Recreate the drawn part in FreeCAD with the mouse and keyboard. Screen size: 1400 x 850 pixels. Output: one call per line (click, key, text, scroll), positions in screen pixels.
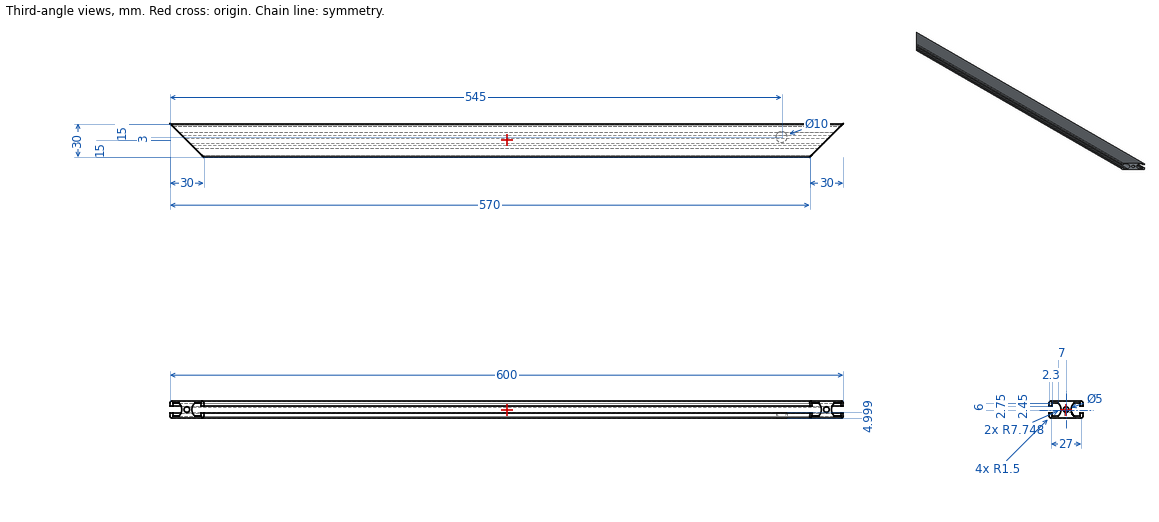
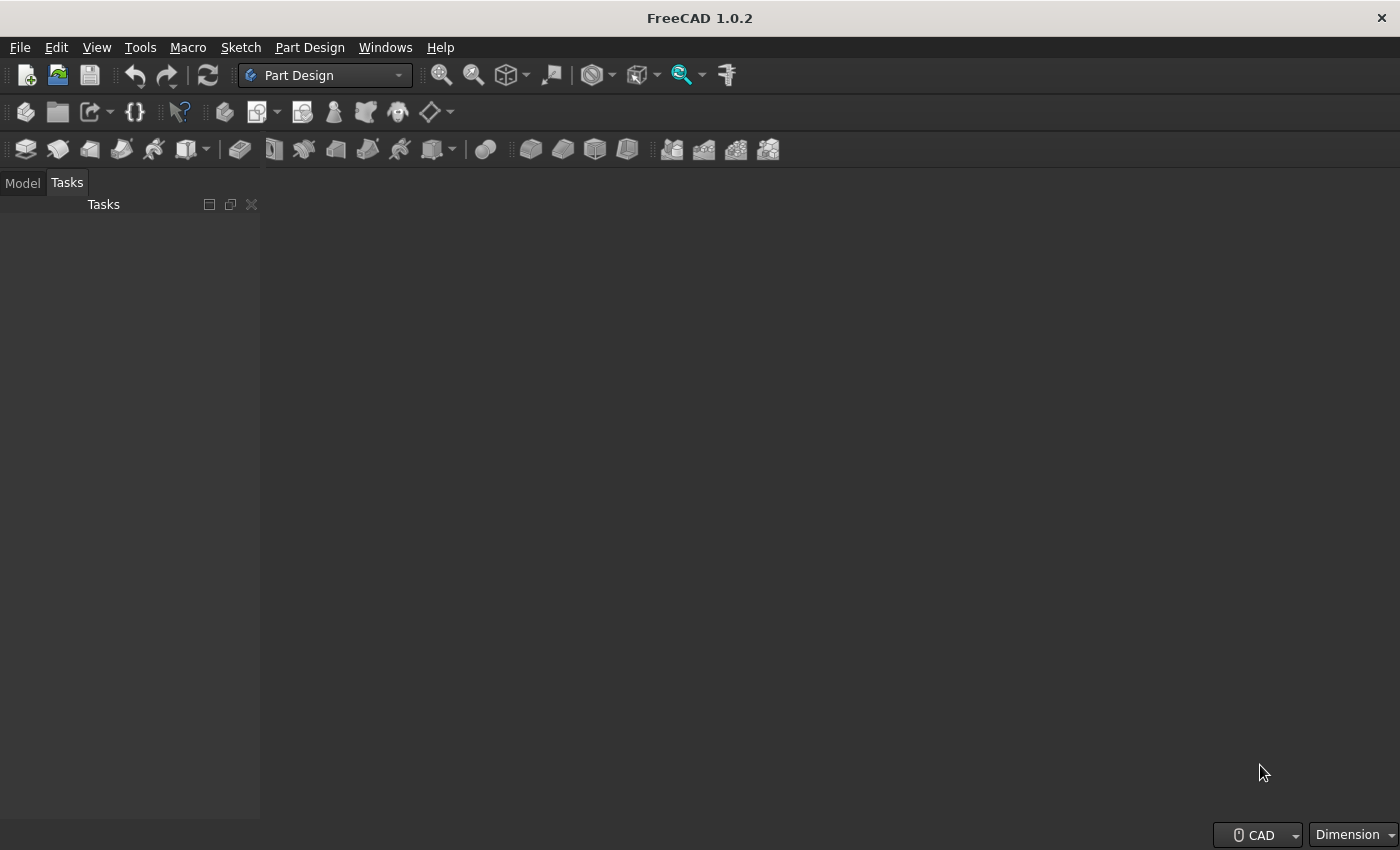
key(ctrl+n)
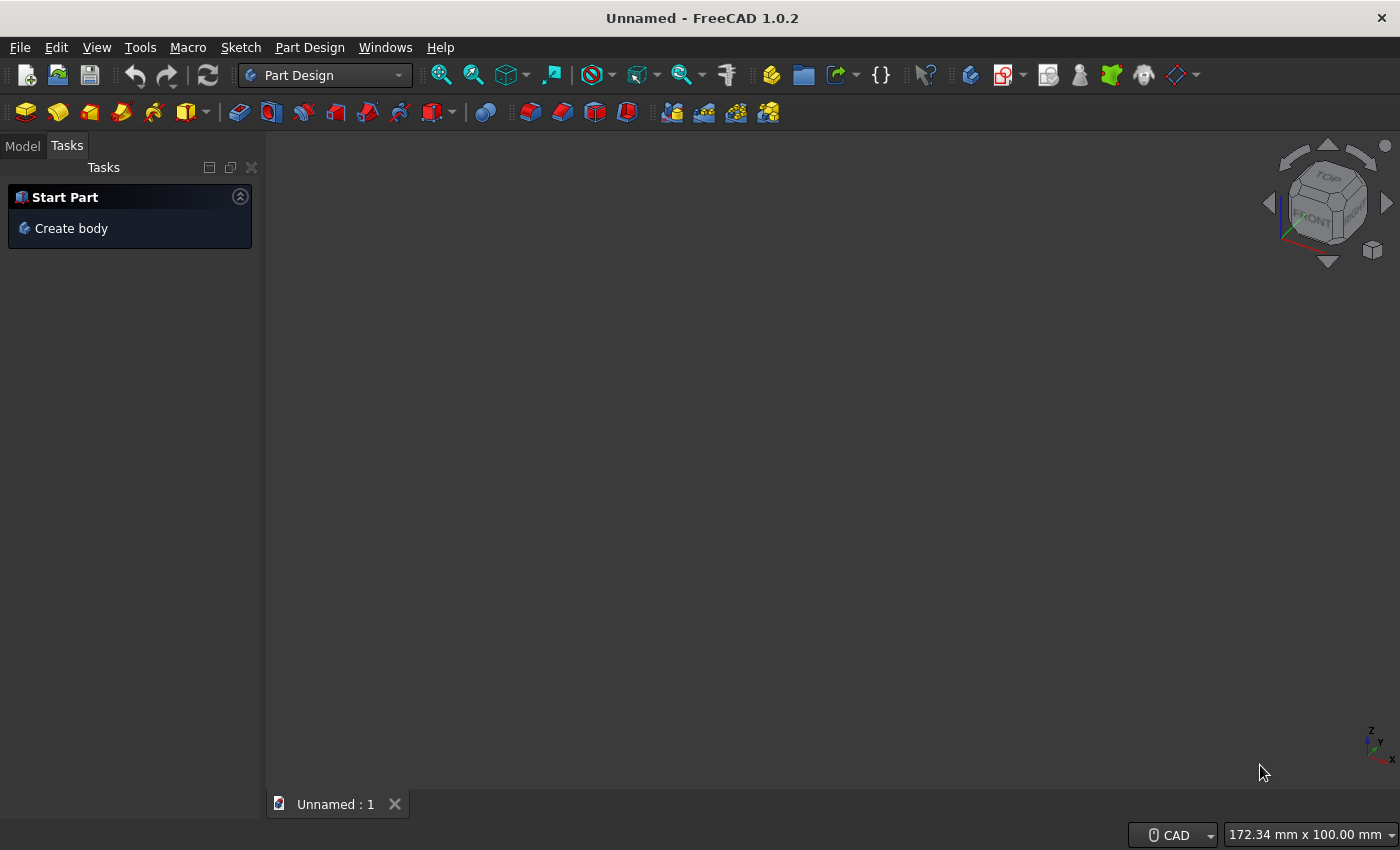
click(972, 76)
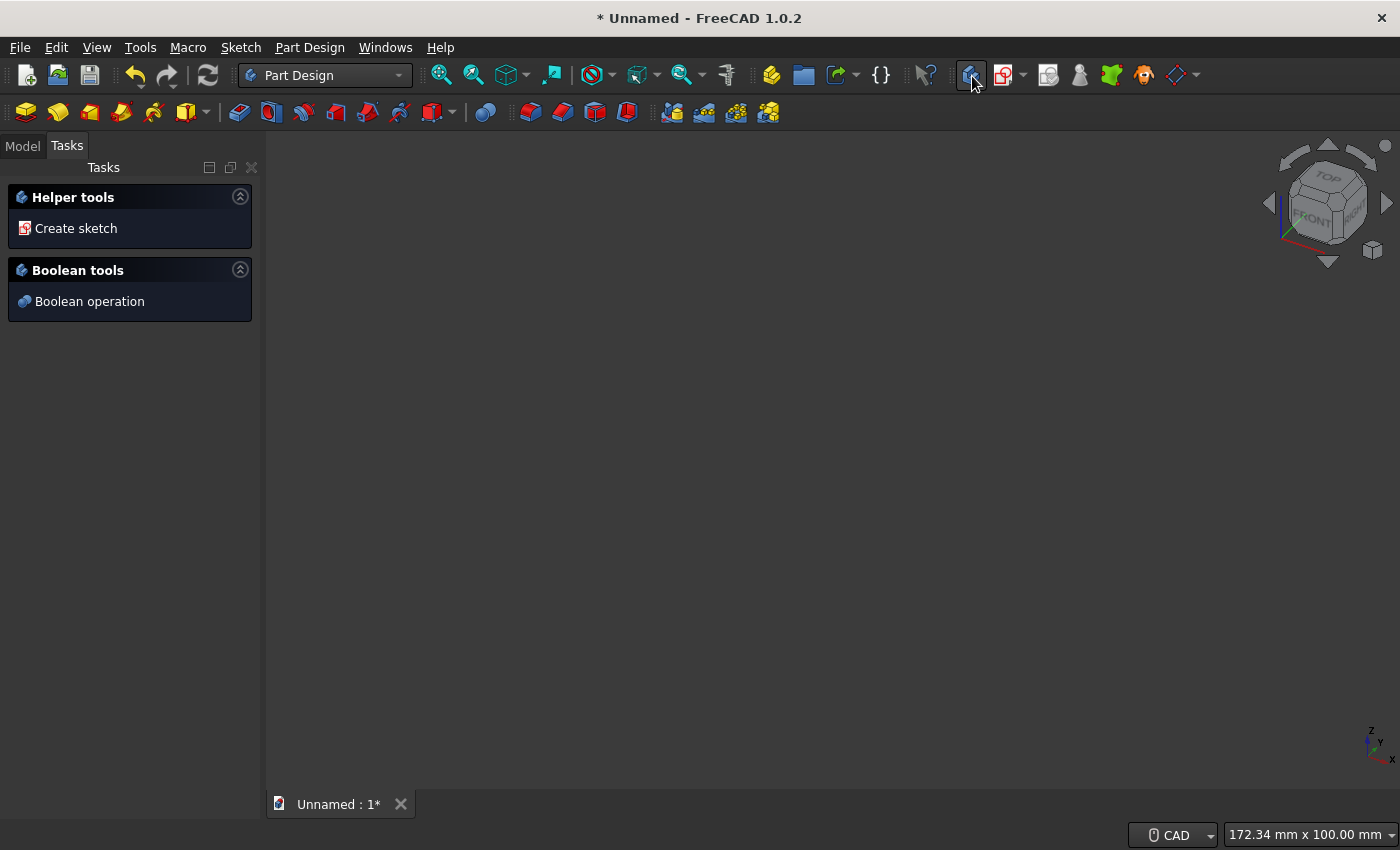
click(23, 145)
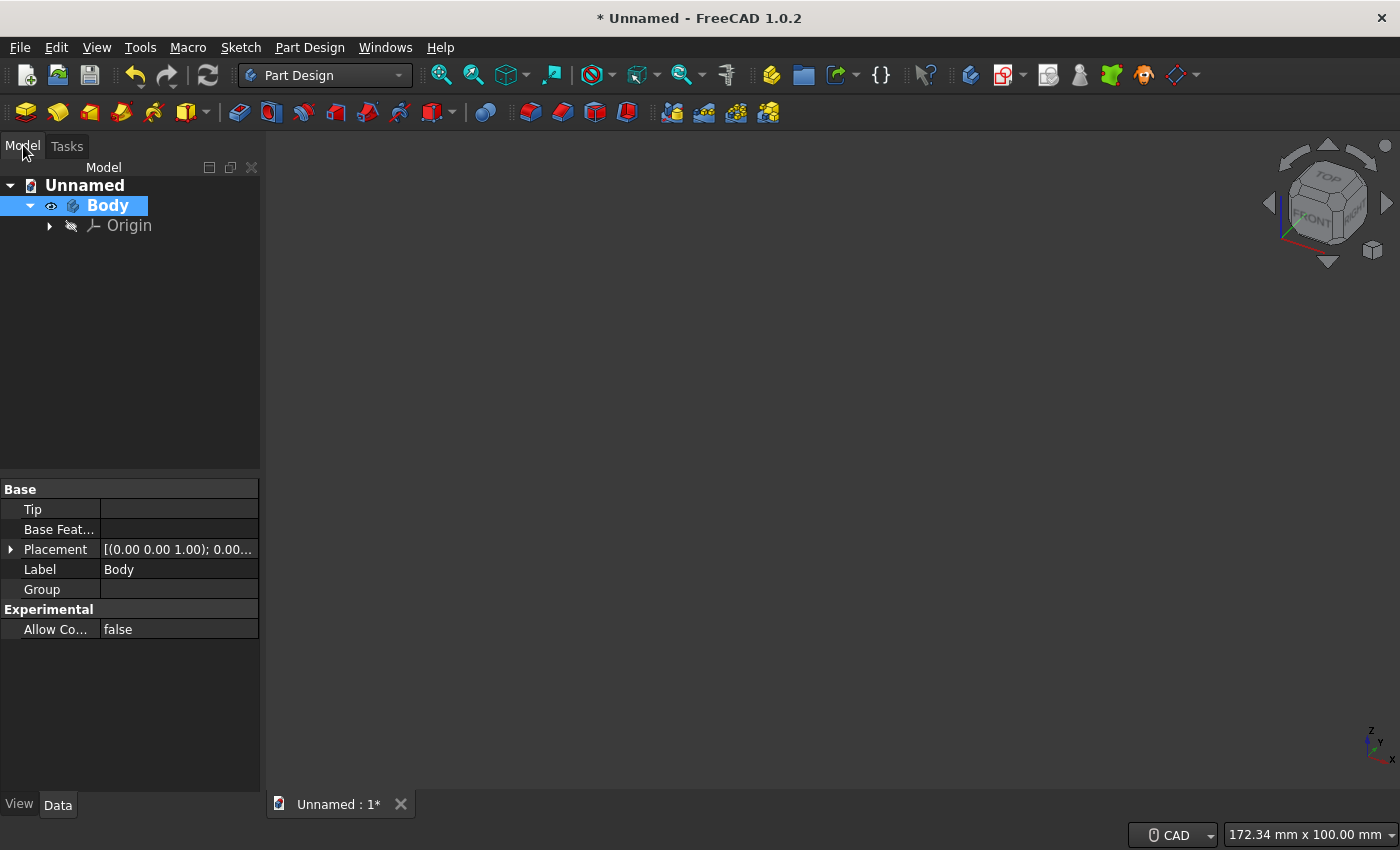
click(50, 226)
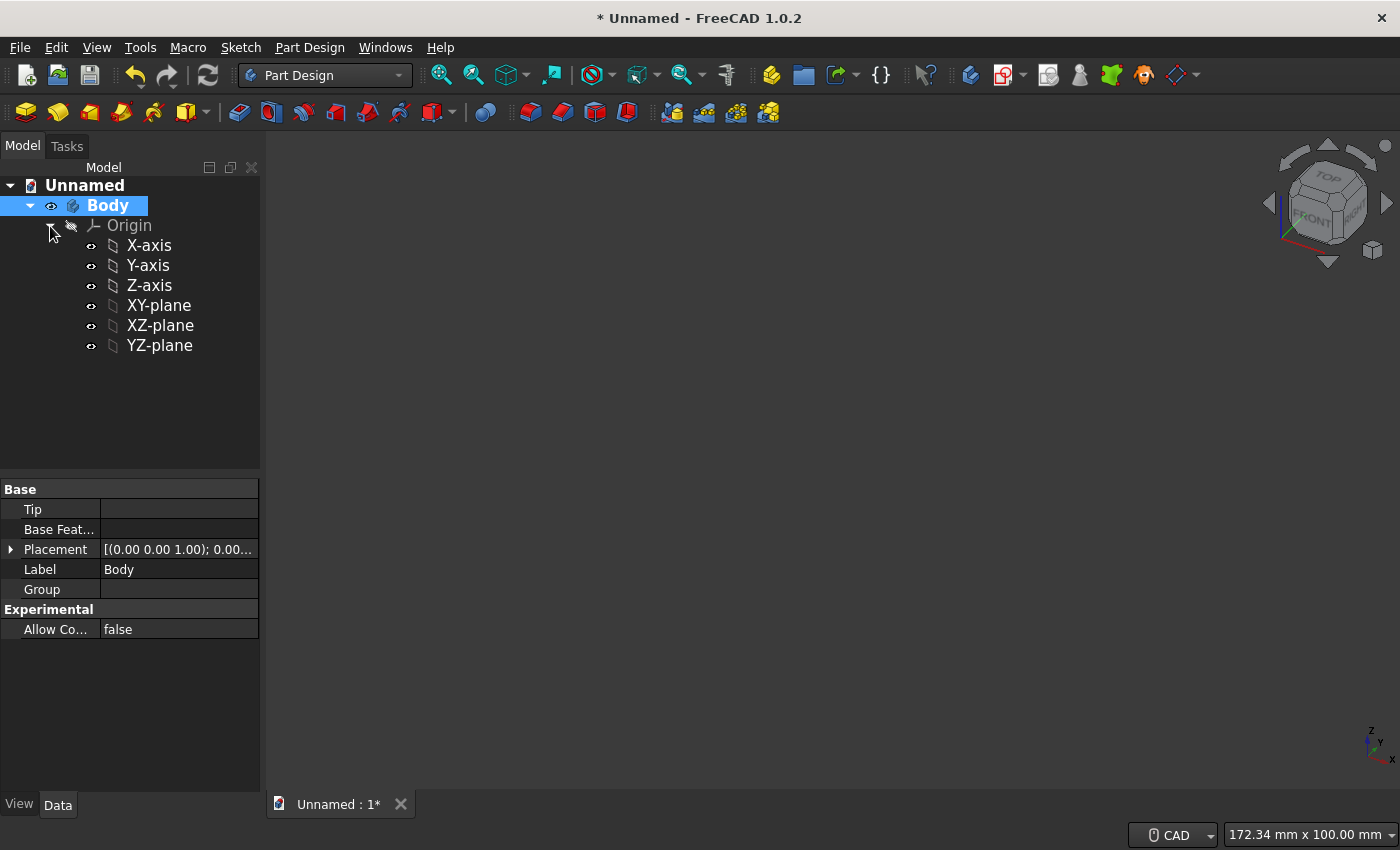
click(136, 346)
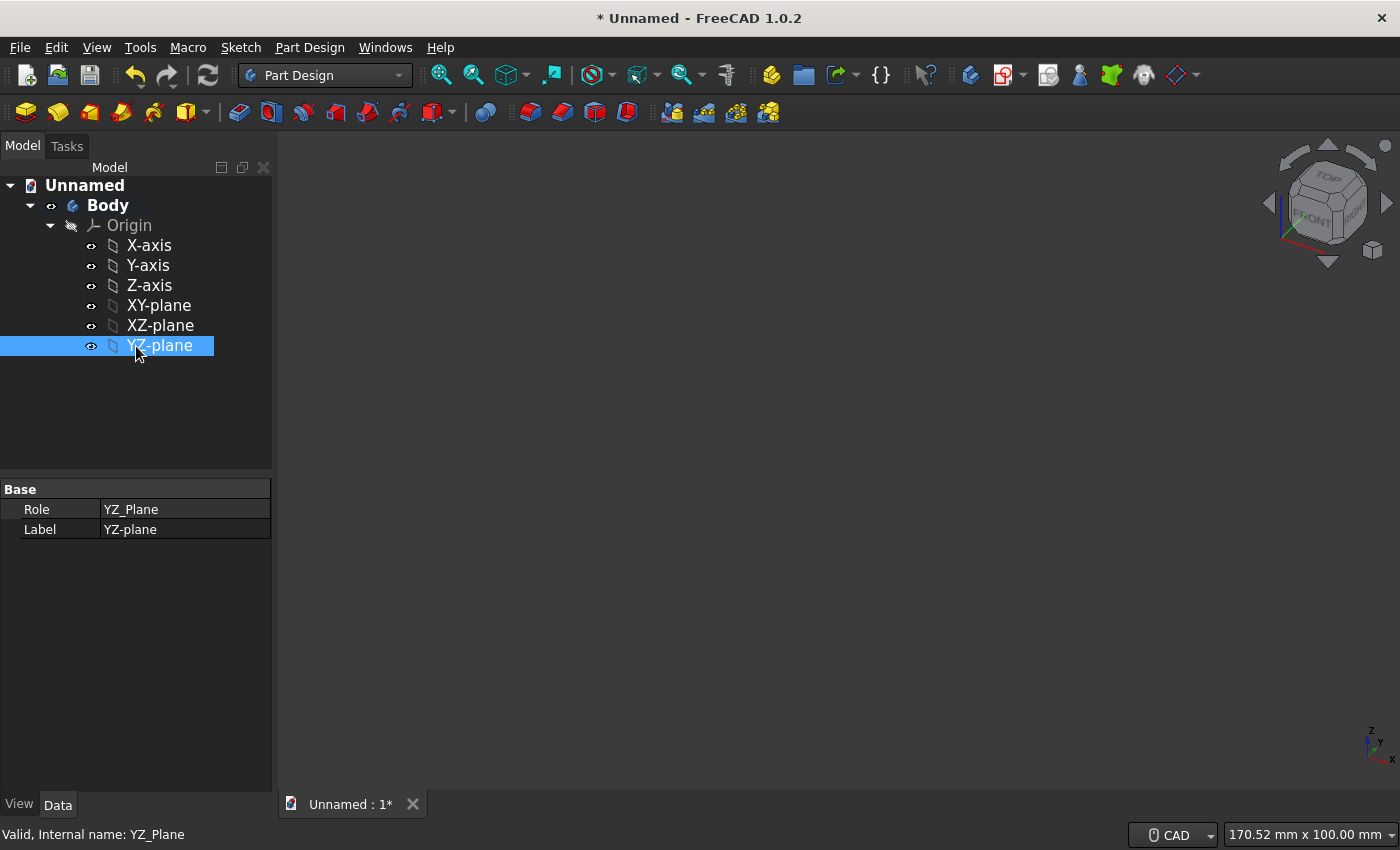
click(1176, 76)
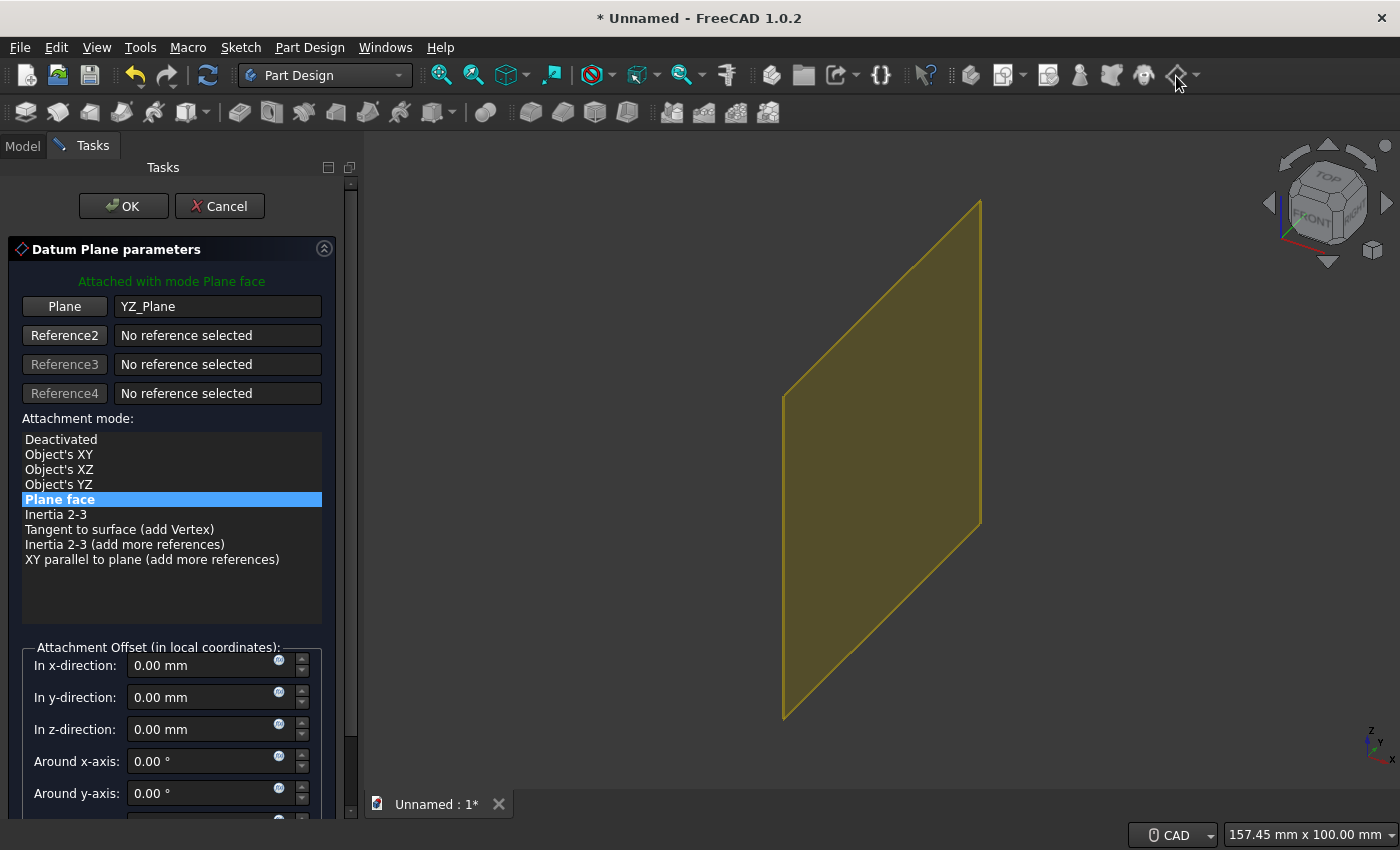
triple_click(210, 729)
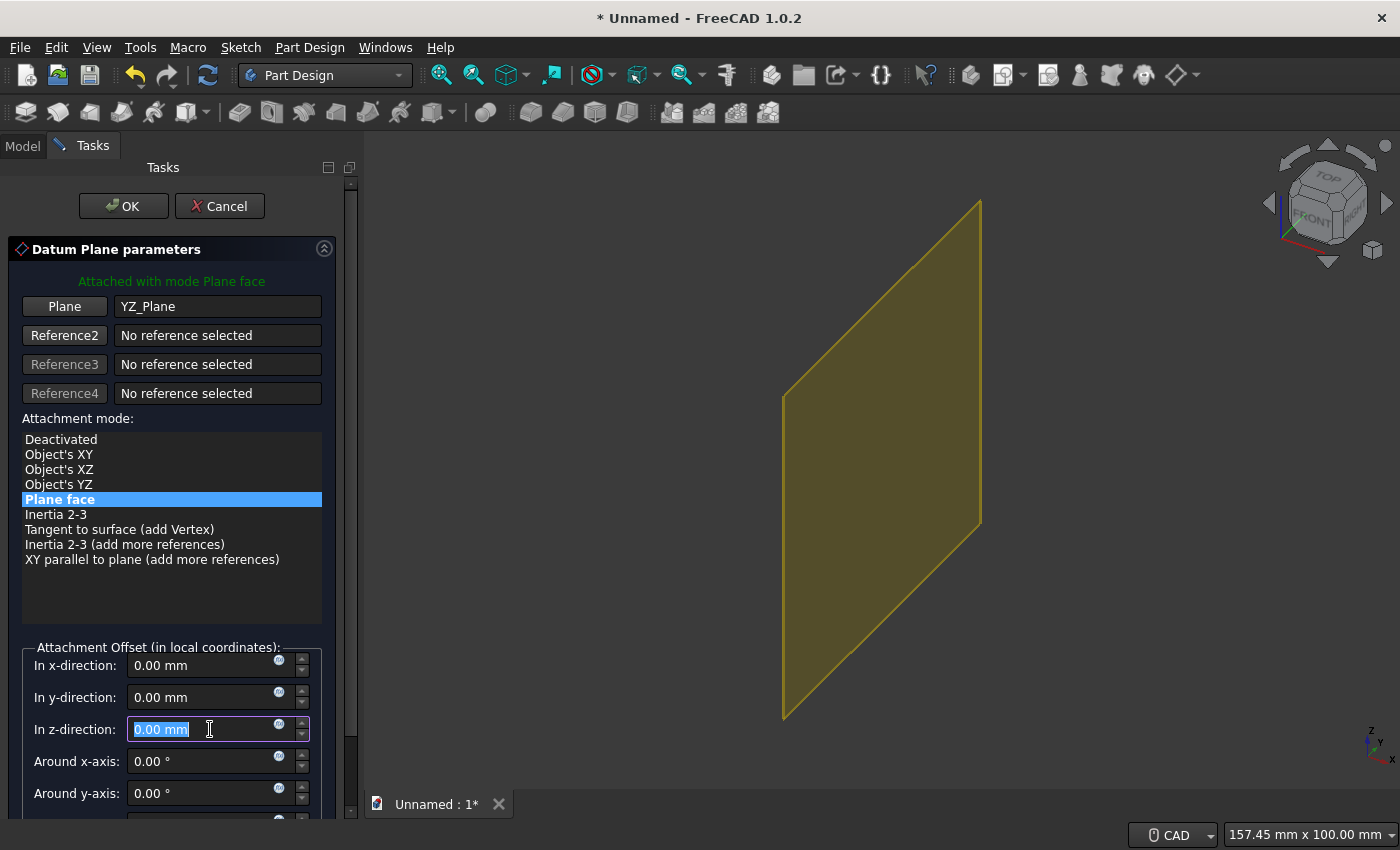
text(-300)
key(Tab)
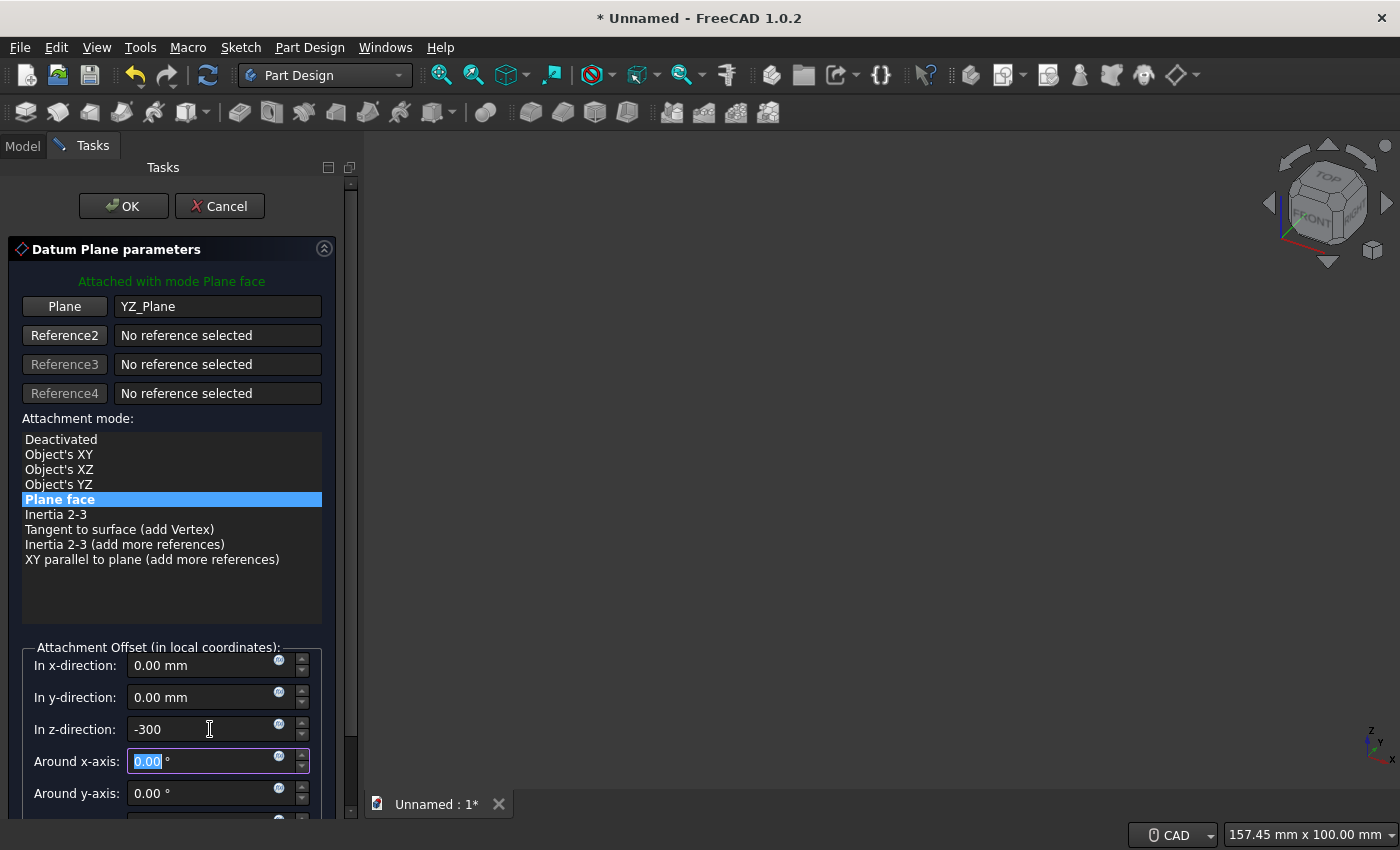
click(124, 206)